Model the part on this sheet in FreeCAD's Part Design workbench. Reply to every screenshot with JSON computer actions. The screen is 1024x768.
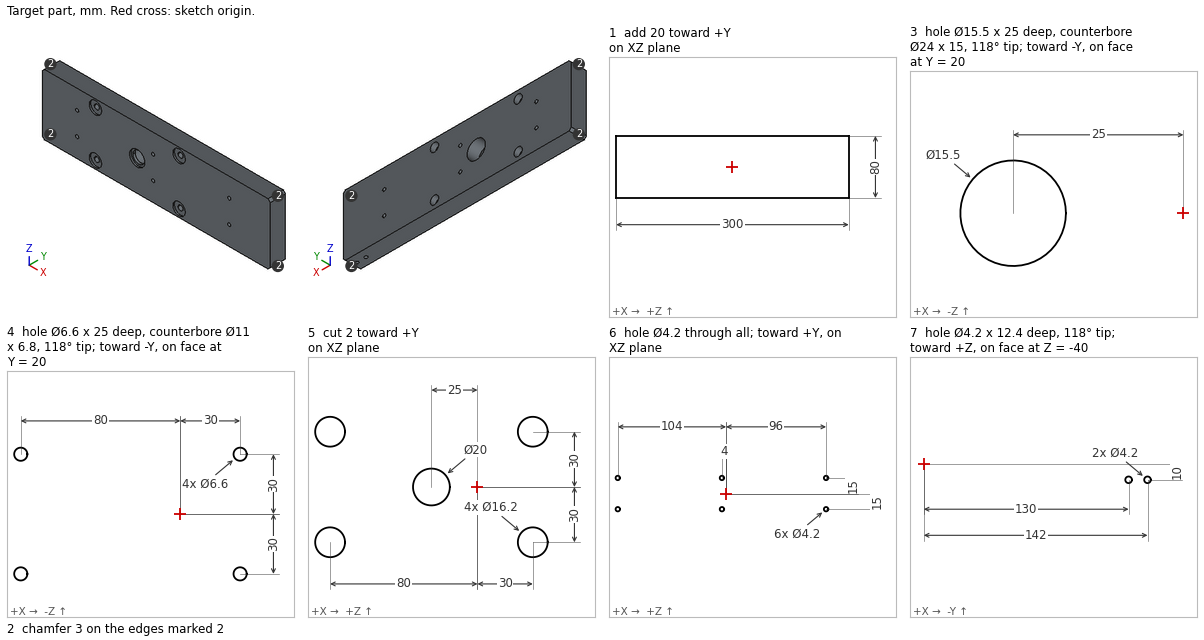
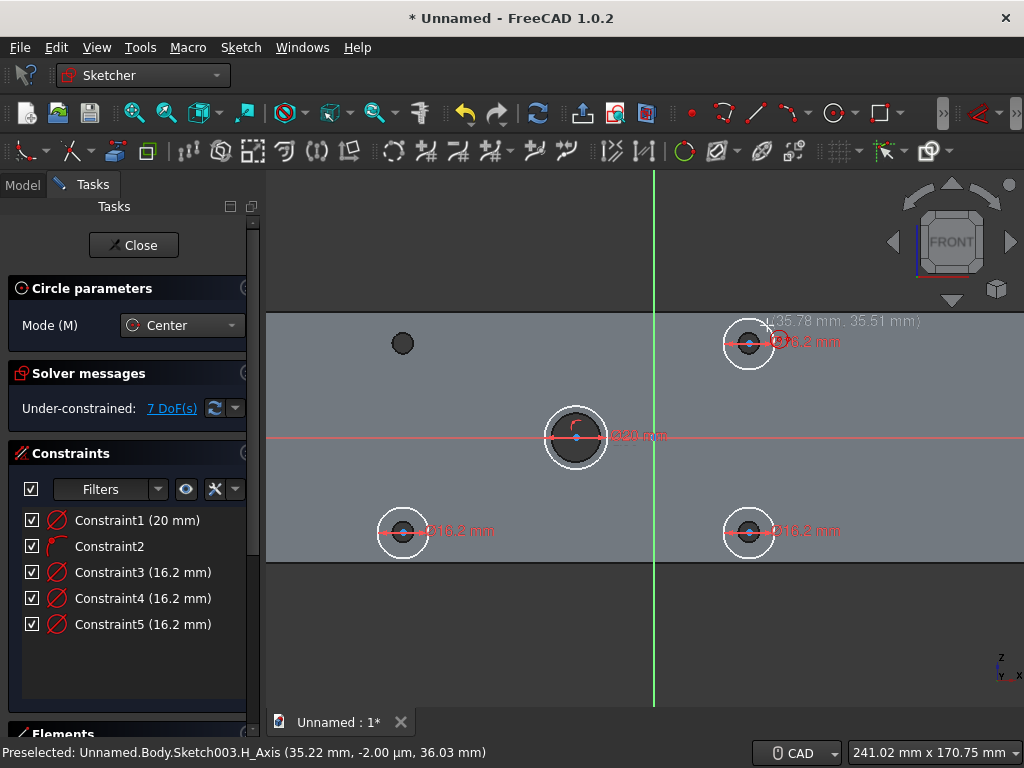
{"action": "left_click", "coordinate": [403, 343]}
{"action": "mouse_move", "coordinate": [421, 325]}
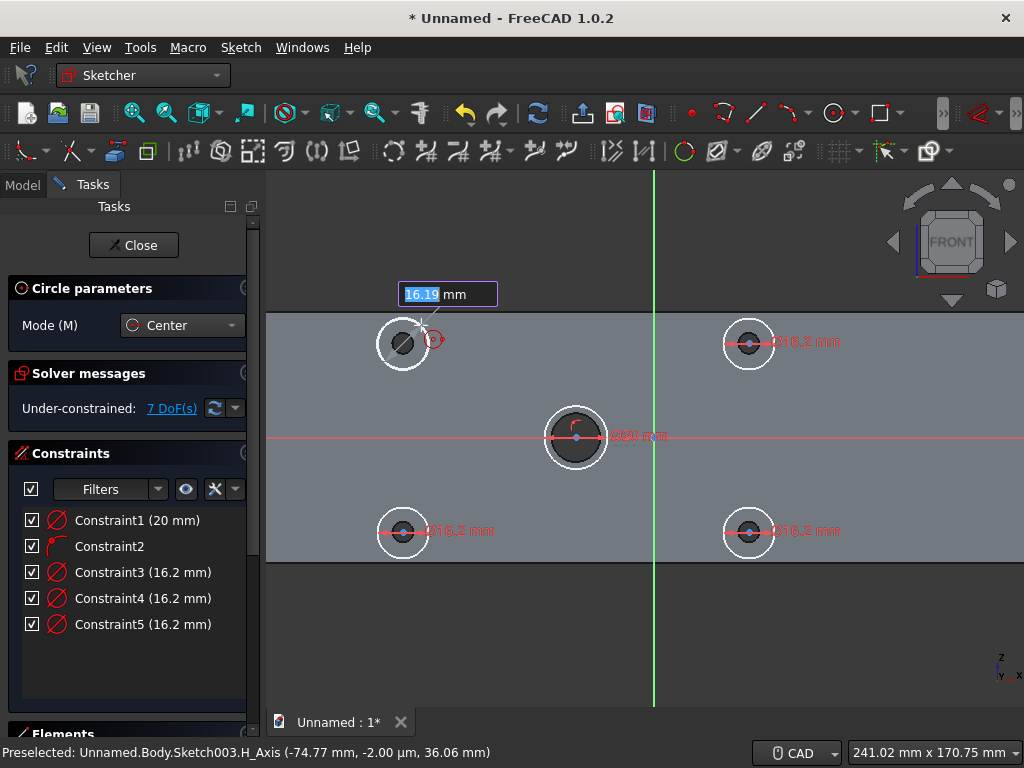
{"action": "type", "text": "16.2"}
{"action": "key", "text": "Return"}
{"action": "key", "text": "Escape"}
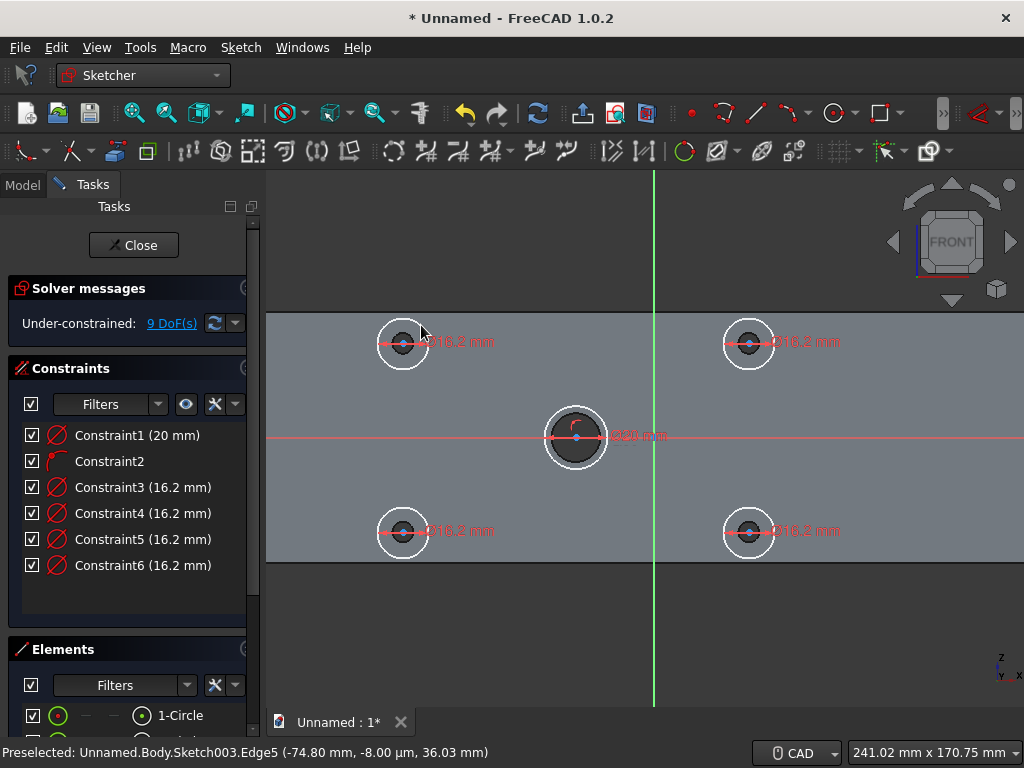
{"action": "left_click", "coordinate": [749, 533]}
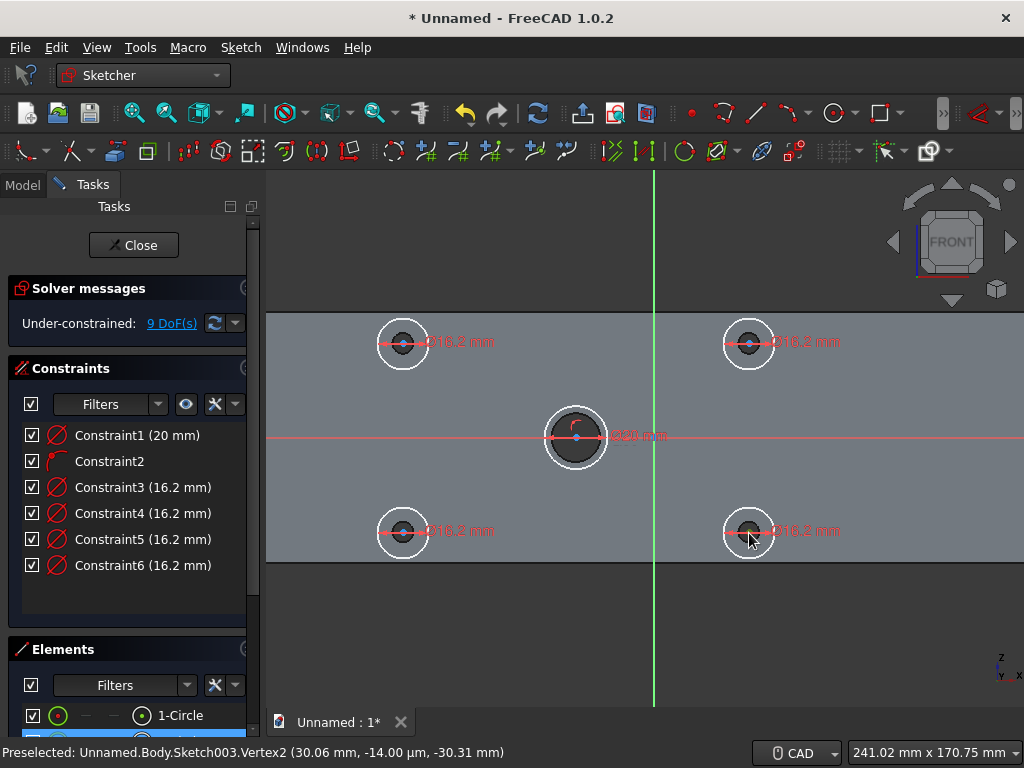
{"action": "left_click", "coordinate": [403, 533]}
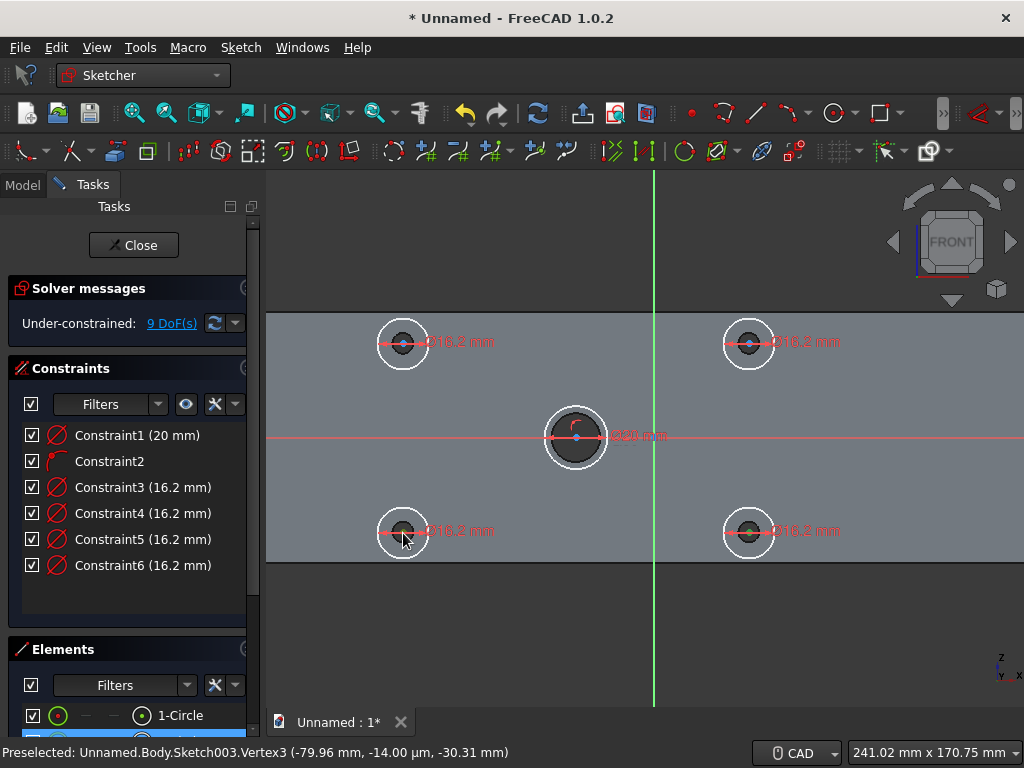
{"action": "key", "text": "h"}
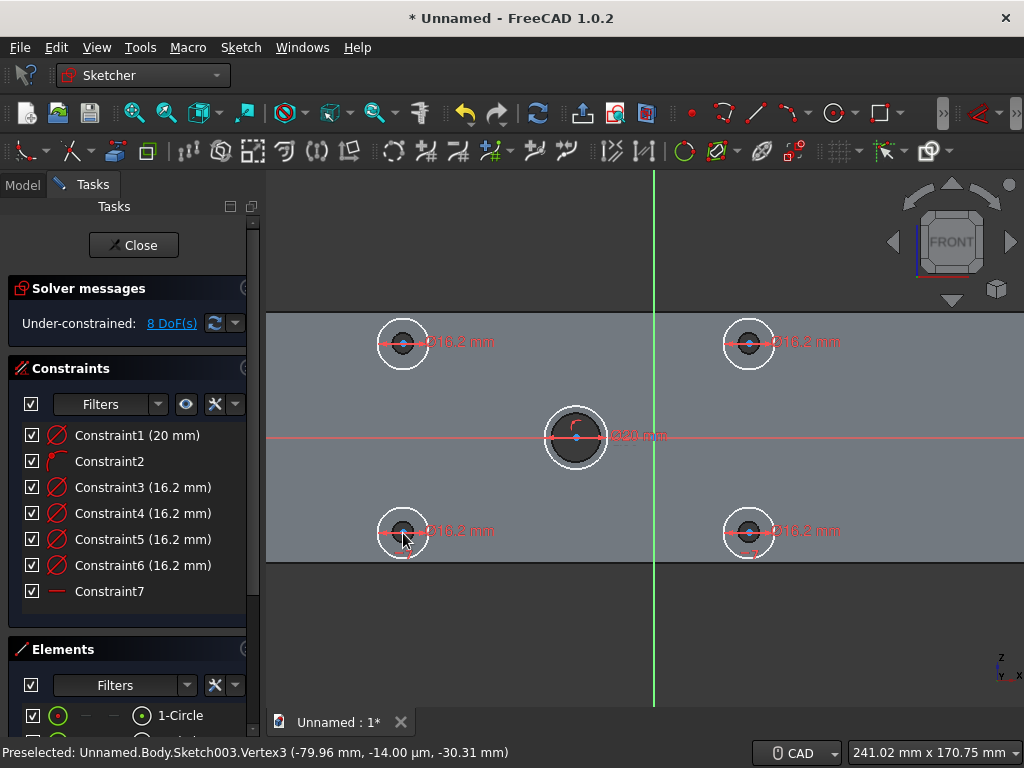
{"action": "left_click", "coordinate": [749, 533]}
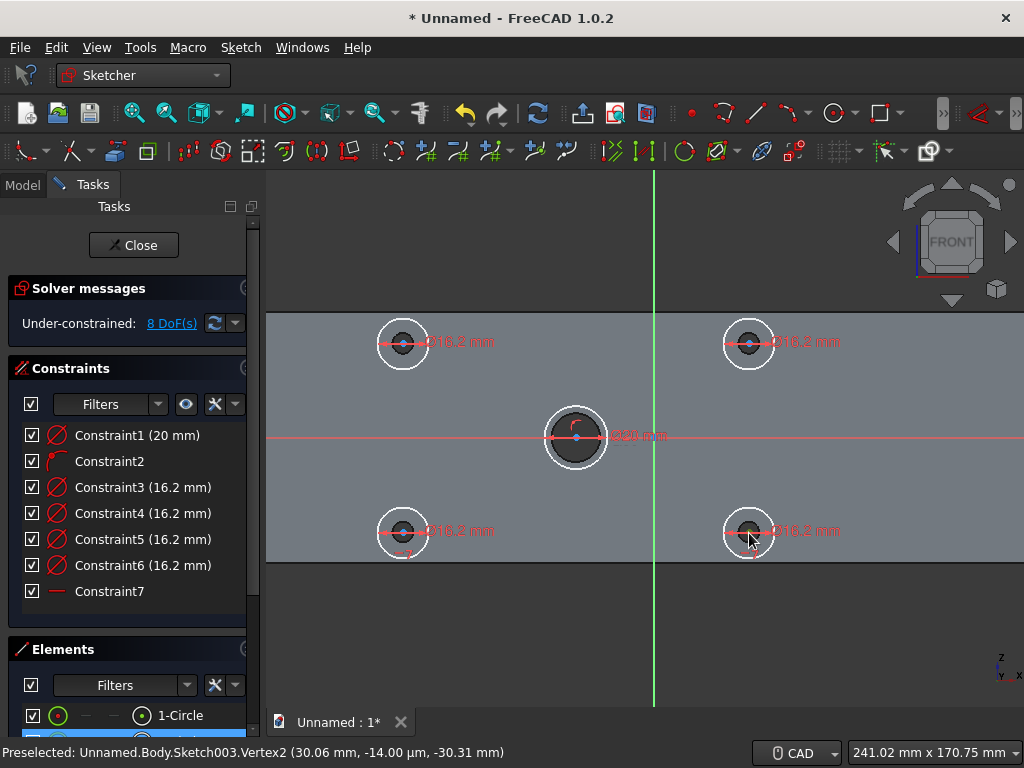
{"action": "left_click", "coordinate": [749, 344]}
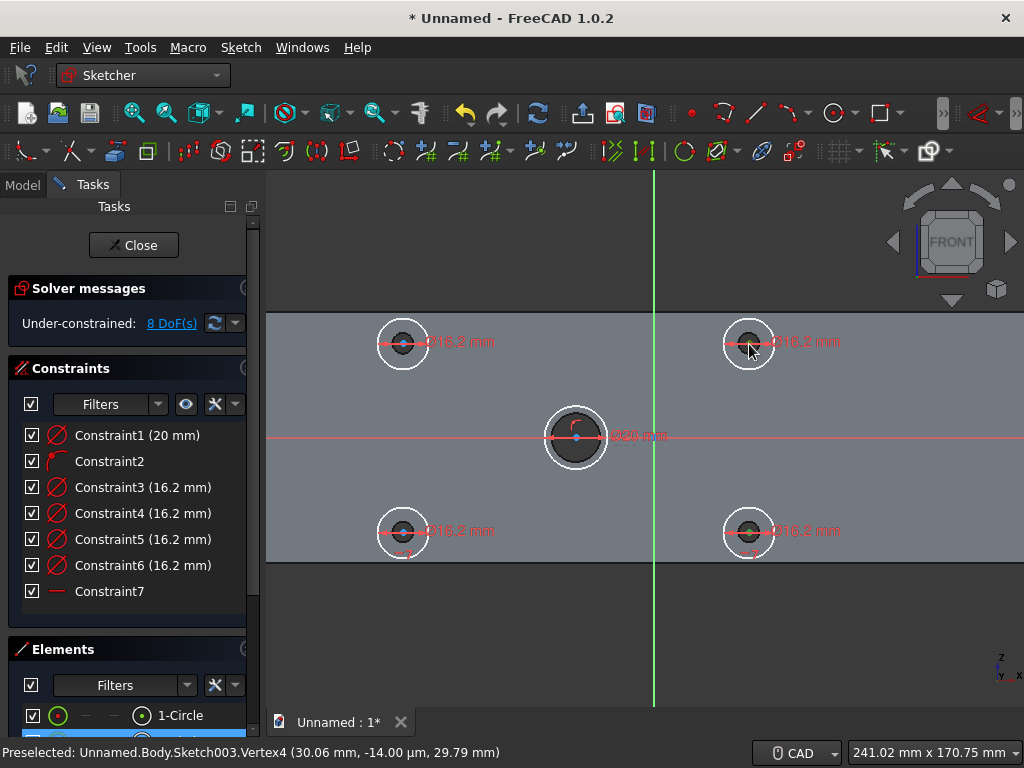
{"action": "key", "text": "v"}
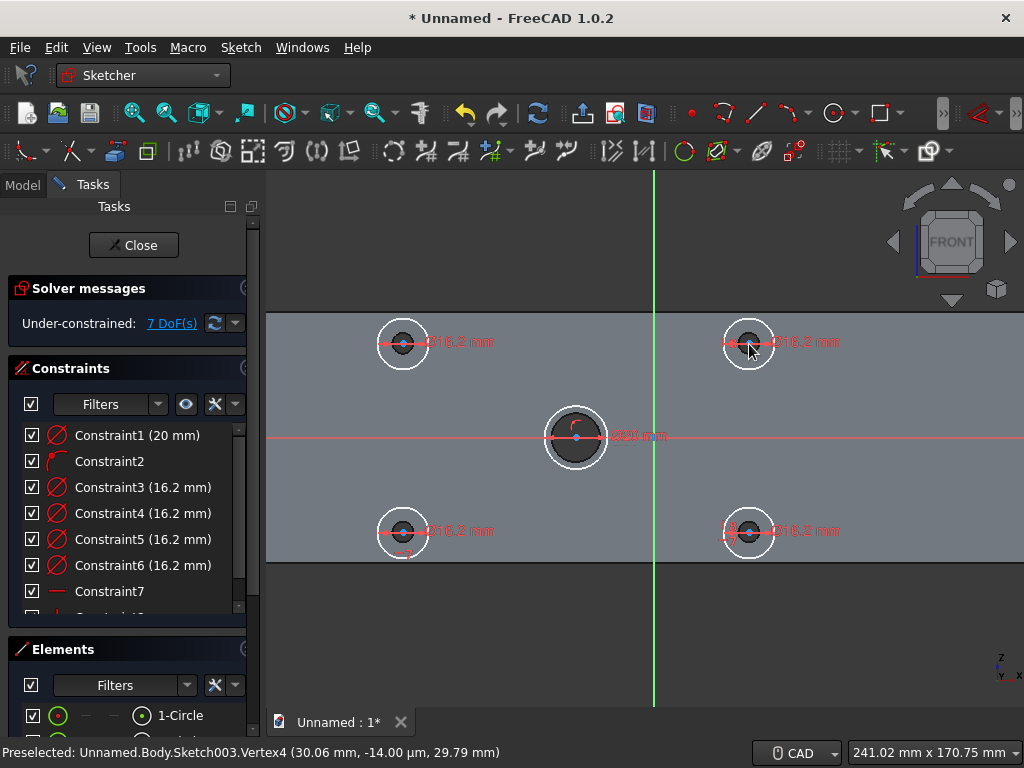
{"action": "left_click", "coordinate": [403, 533]}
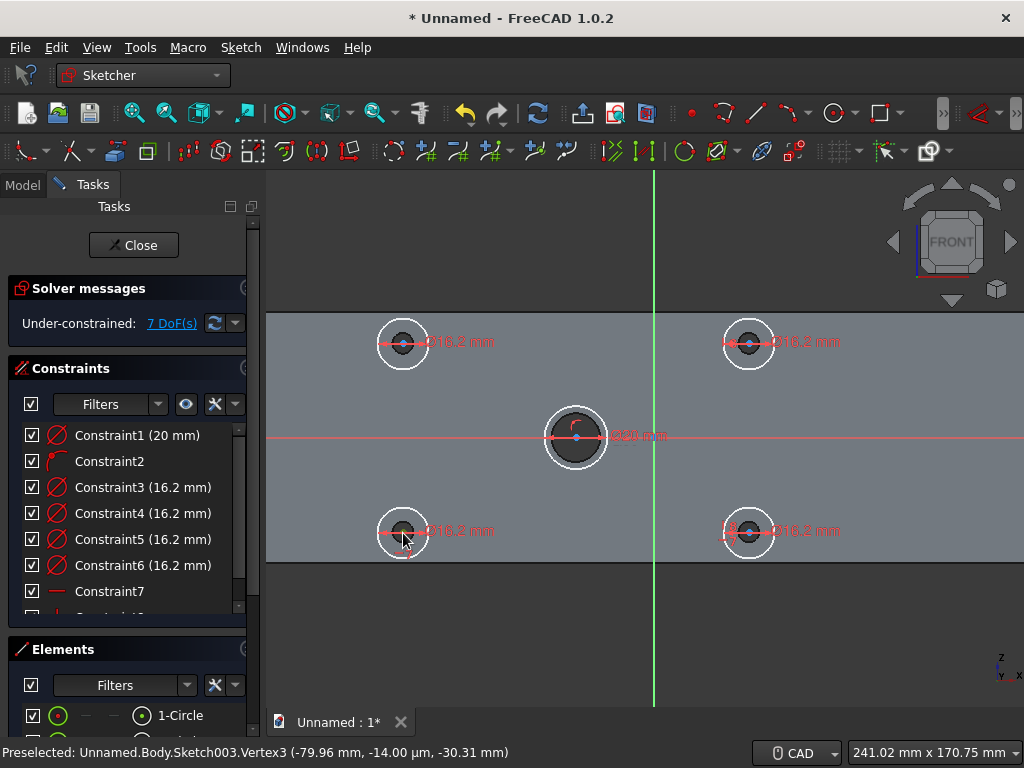
{"action": "left_click", "coordinate": [403, 344]}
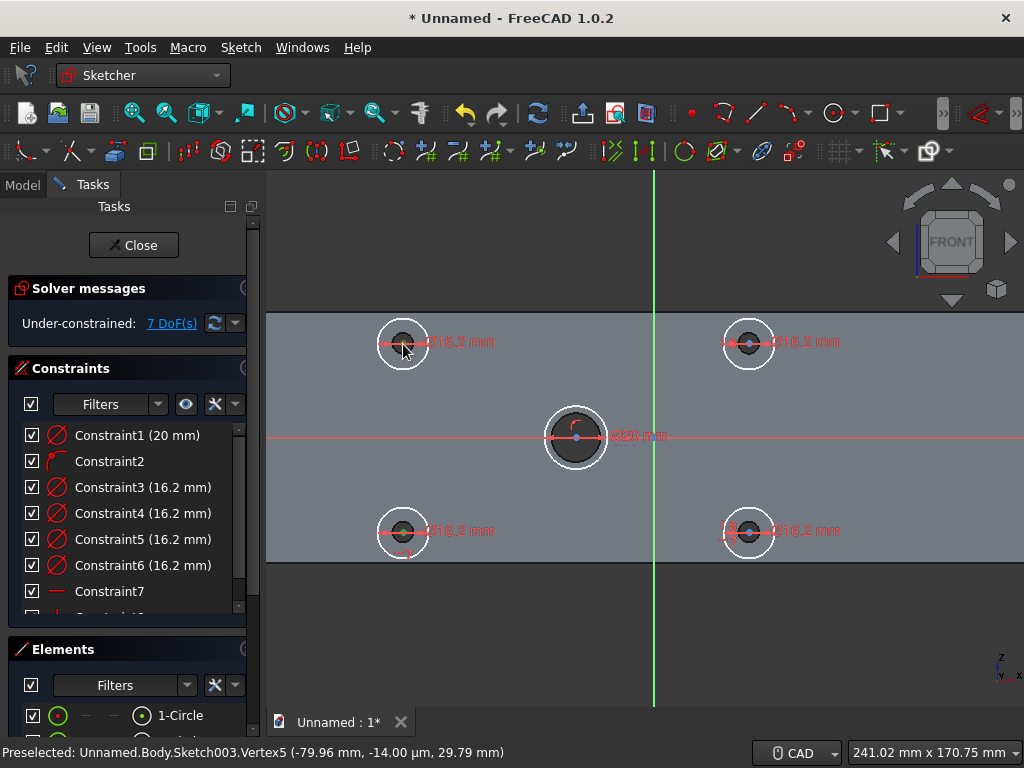
{"action": "key", "text": "v"}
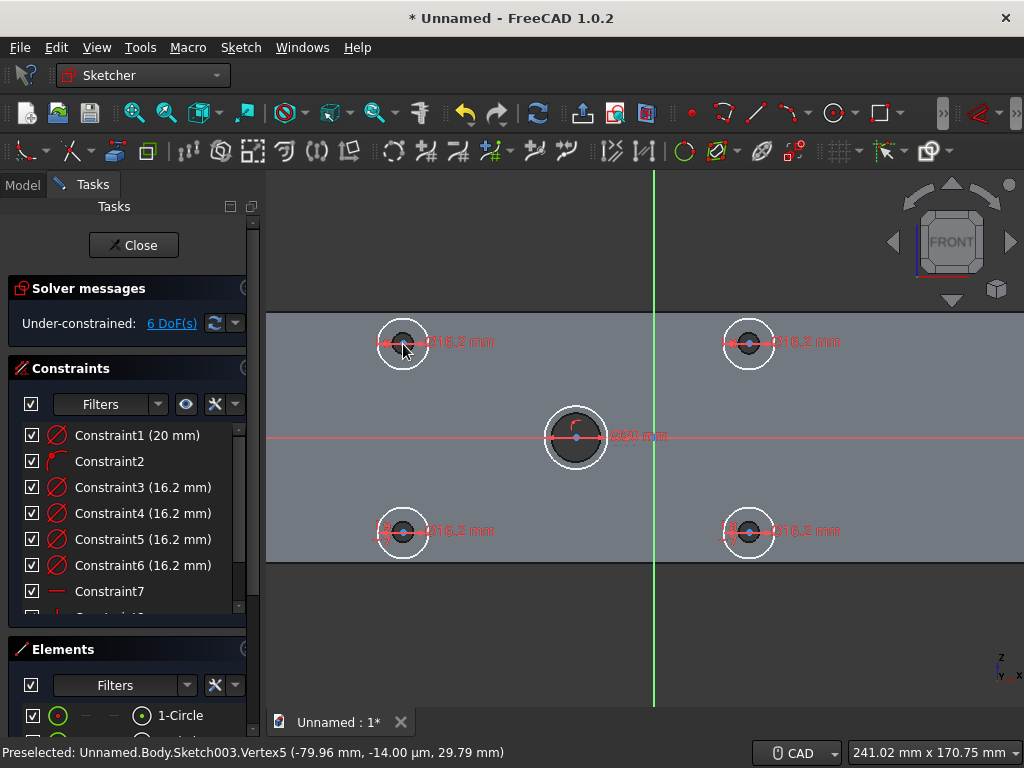
{"action": "left_click", "coordinate": [749, 344]}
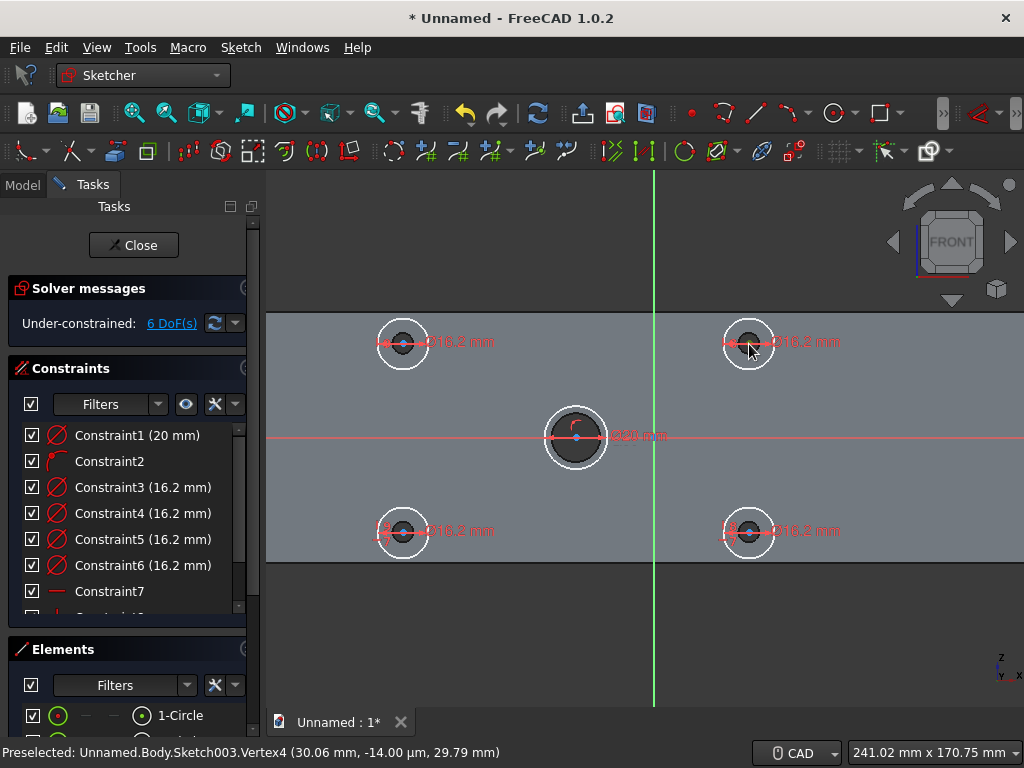
{"action": "left_click", "coordinate": [403, 344]}